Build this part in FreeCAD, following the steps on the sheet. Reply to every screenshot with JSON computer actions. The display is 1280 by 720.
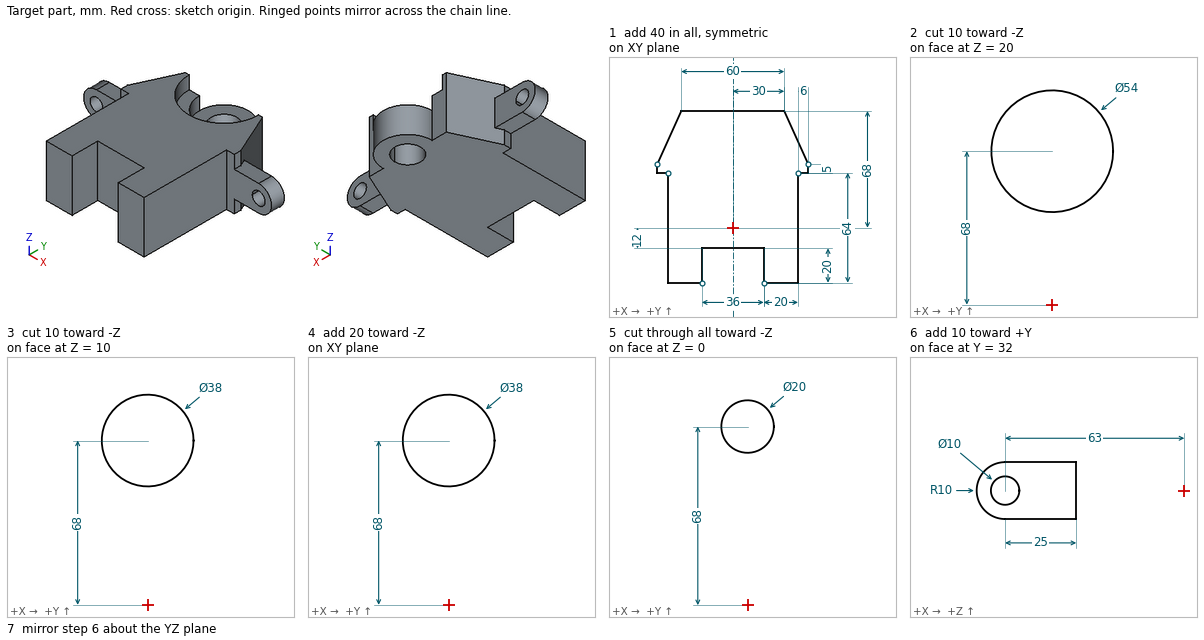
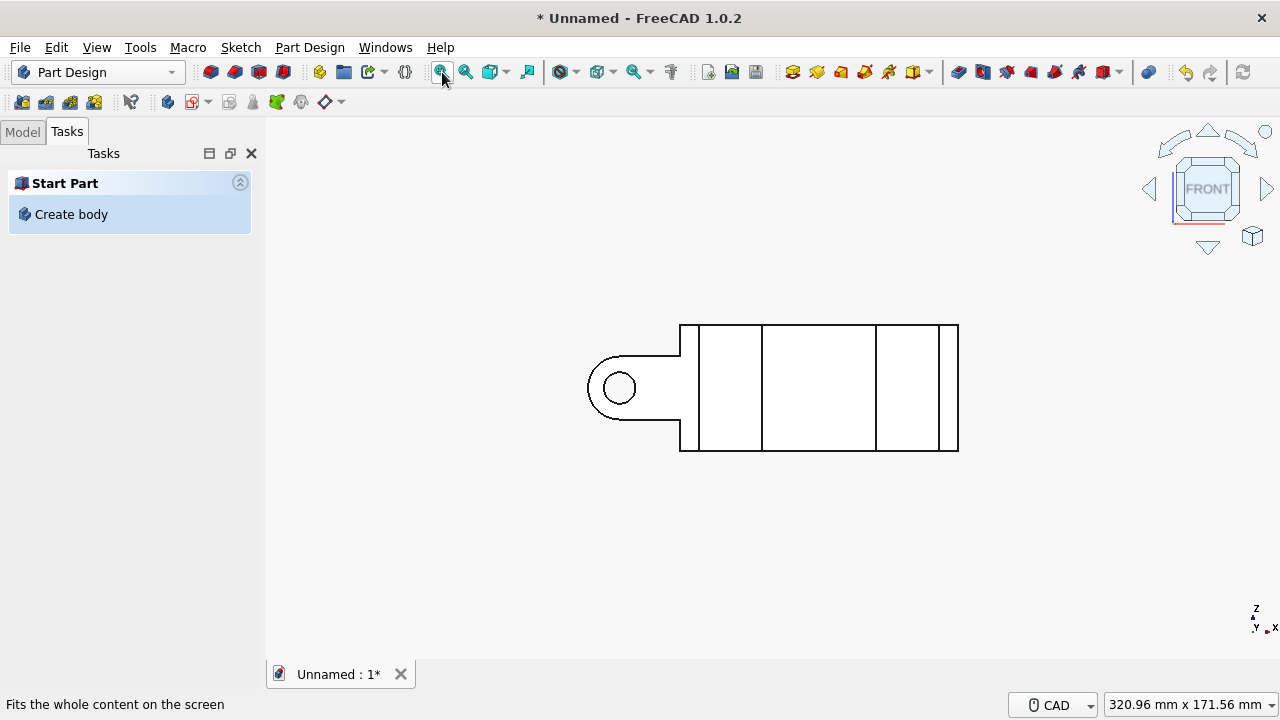
{"action": "left_click", "coordinate": [23, 131]}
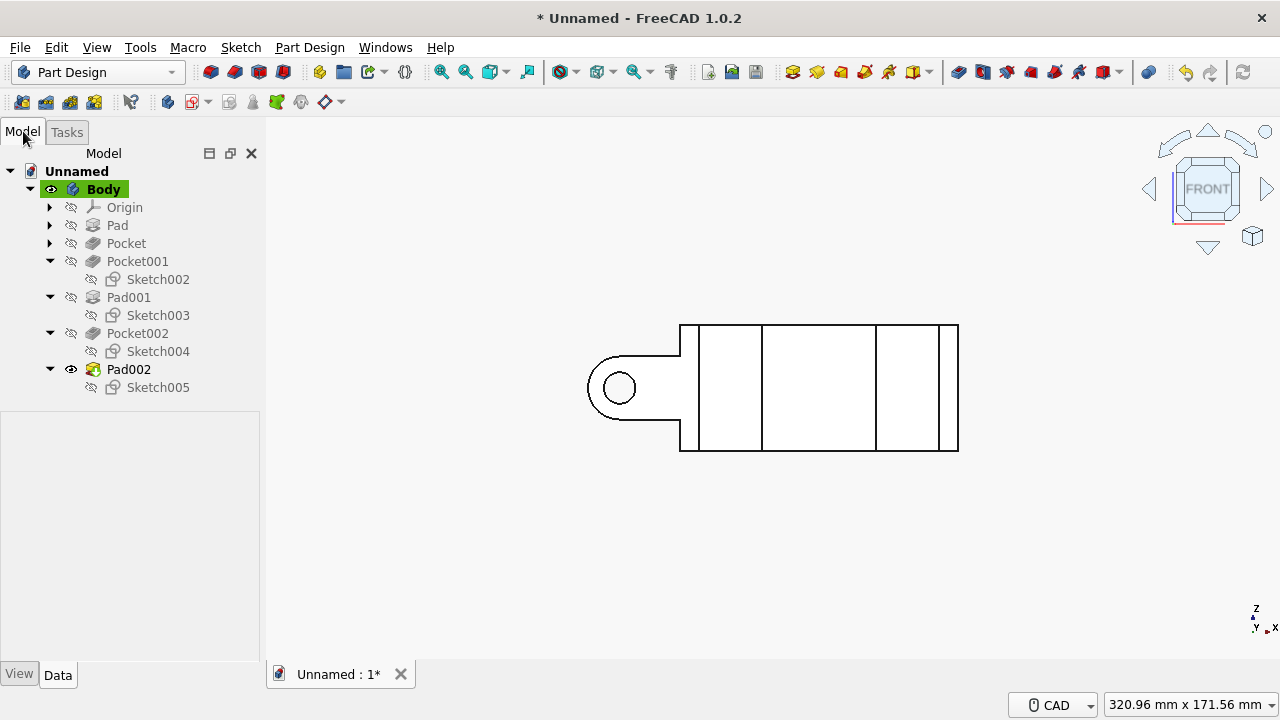
{"action": "left_click", "coordinate": [116, 369]}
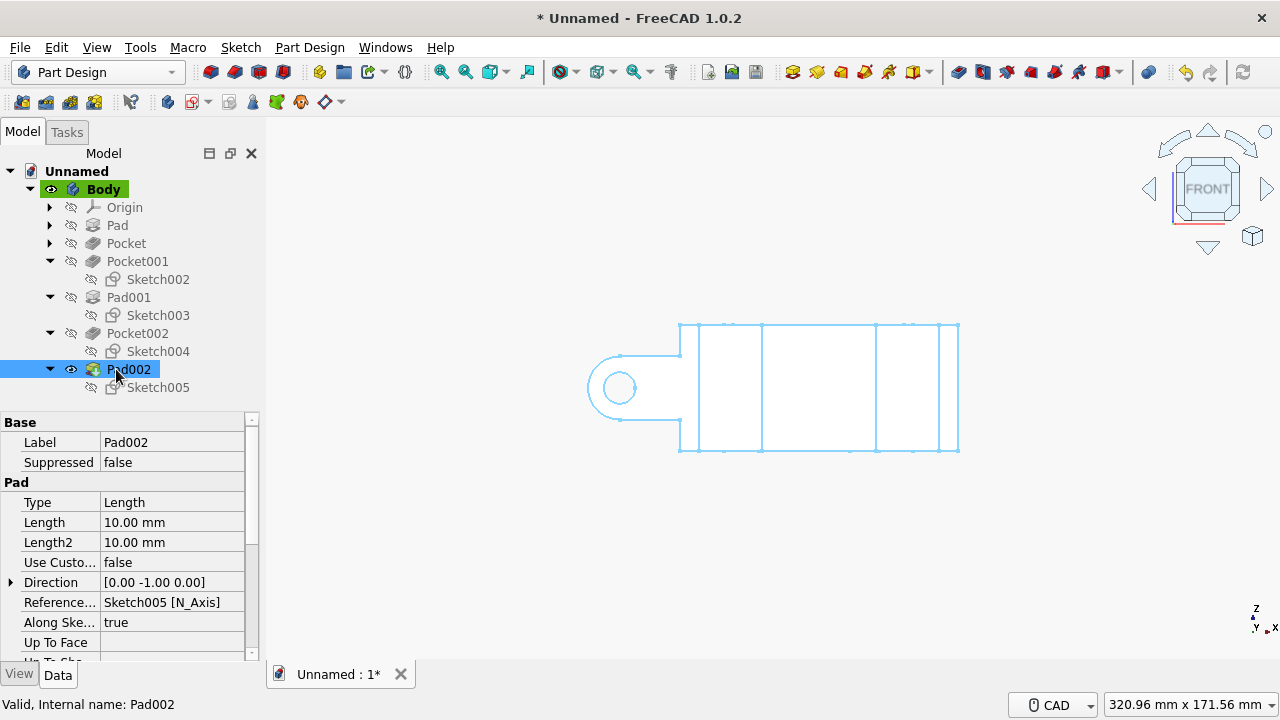
{"action": "left_click", "coordinate": [22, 102]}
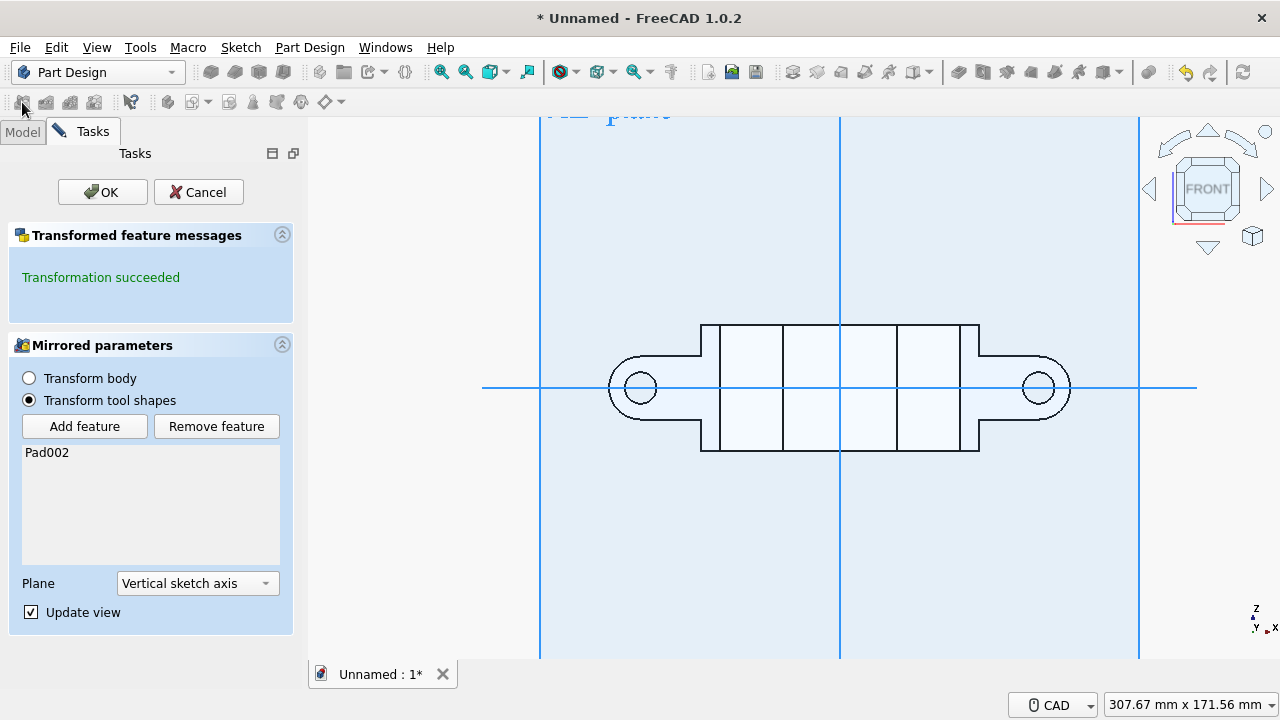
{"action": "left_click", "coordinate": [198, 584]}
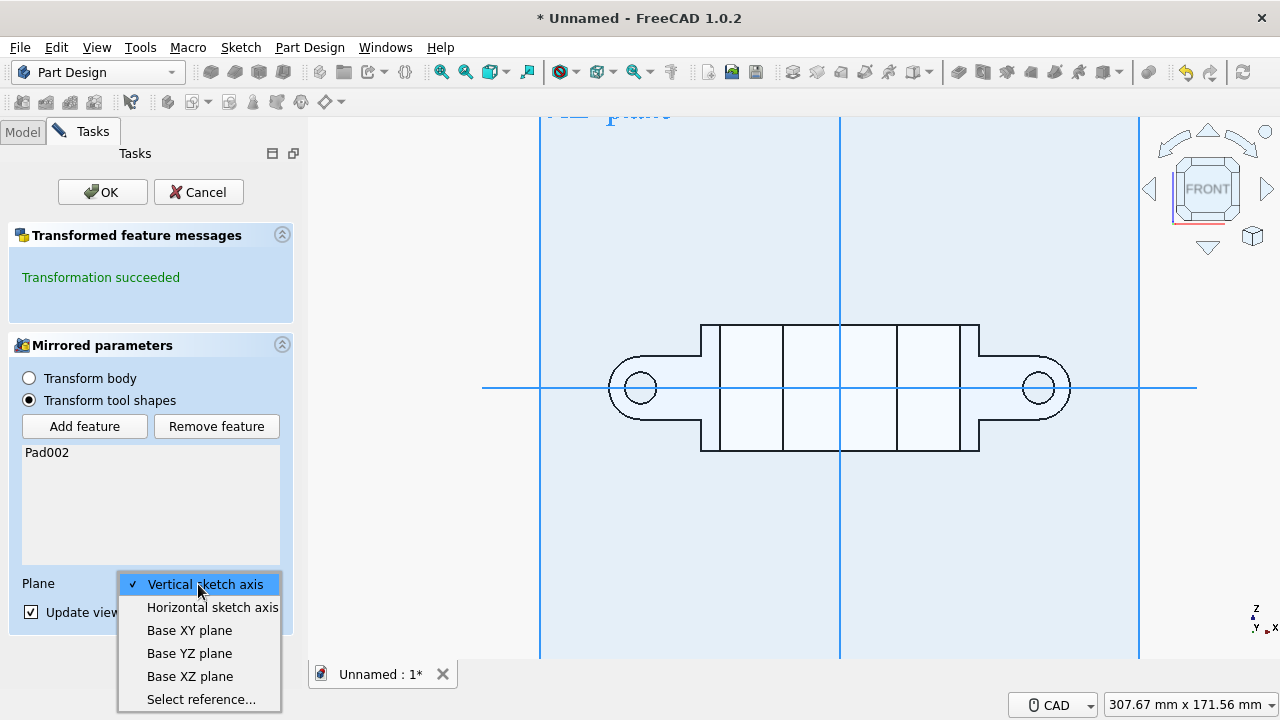
{"action": "left_click", "coordinate": [198, 654]}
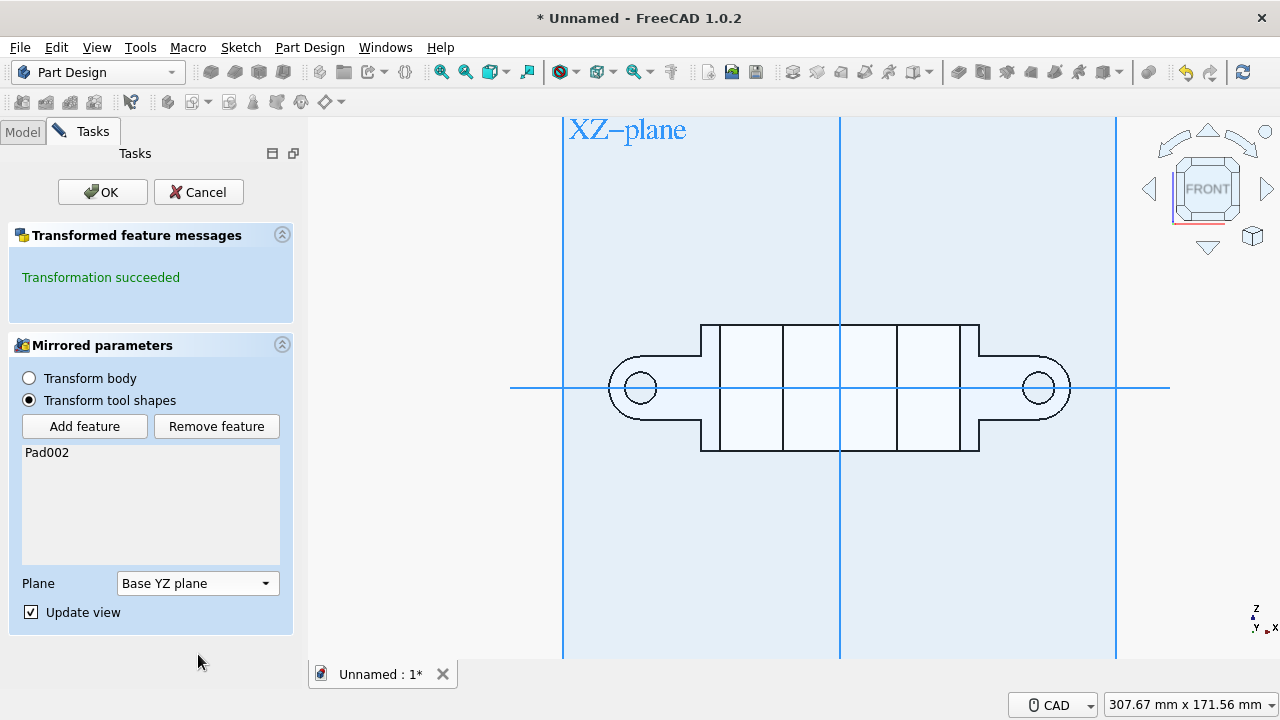
{"action": "left_click", "coordinate": [103, 192]}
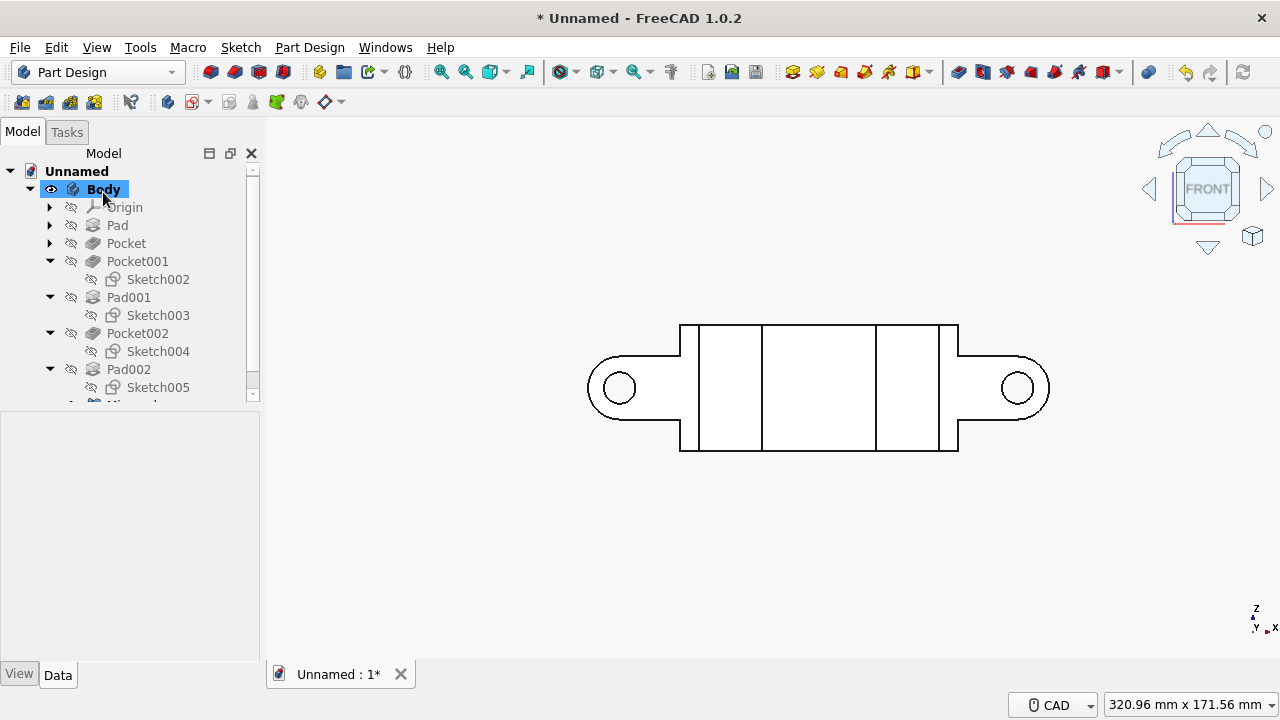
{"action": "key", "text": "0"}